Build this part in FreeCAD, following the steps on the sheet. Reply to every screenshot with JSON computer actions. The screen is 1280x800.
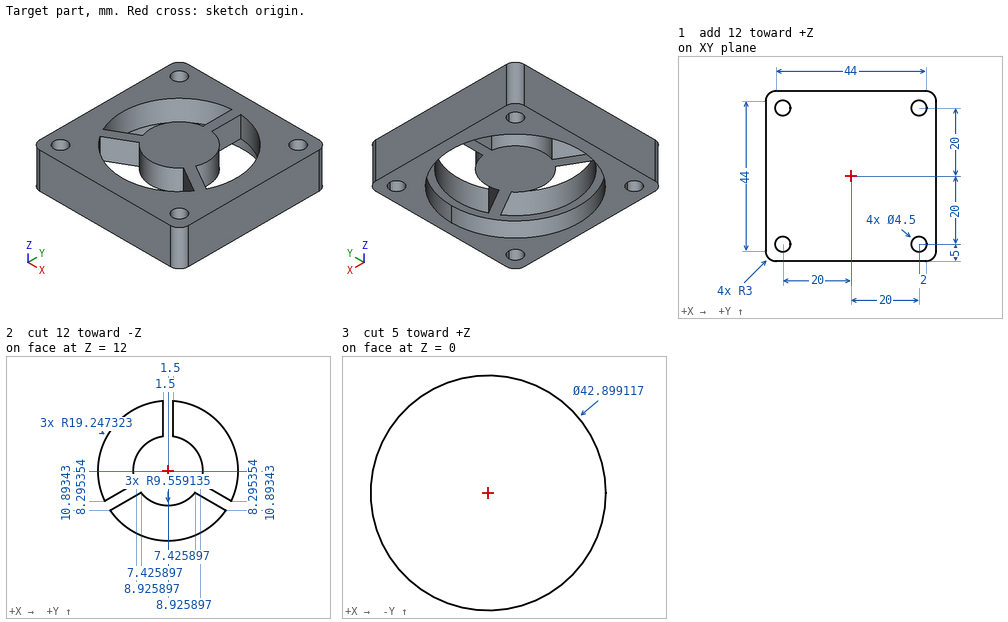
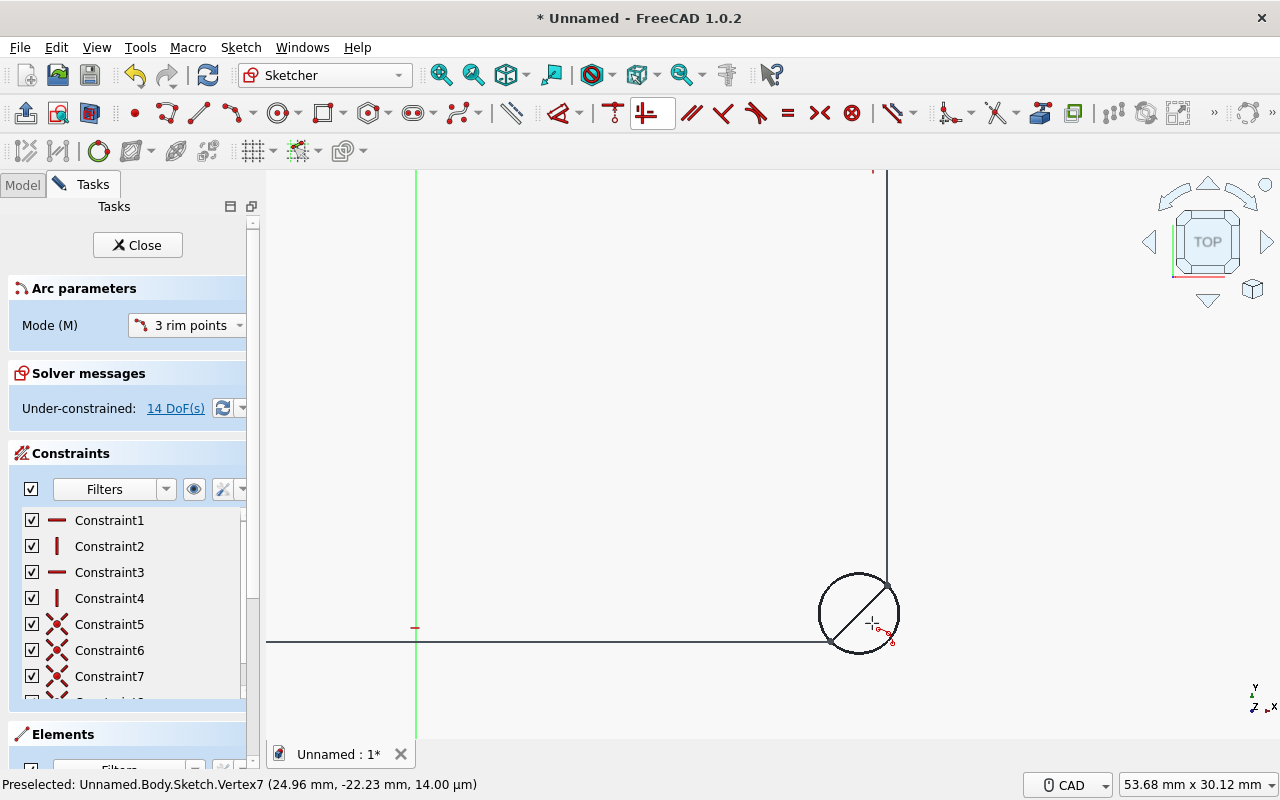
{"action": "left_click", "coordinate": [871, 621]}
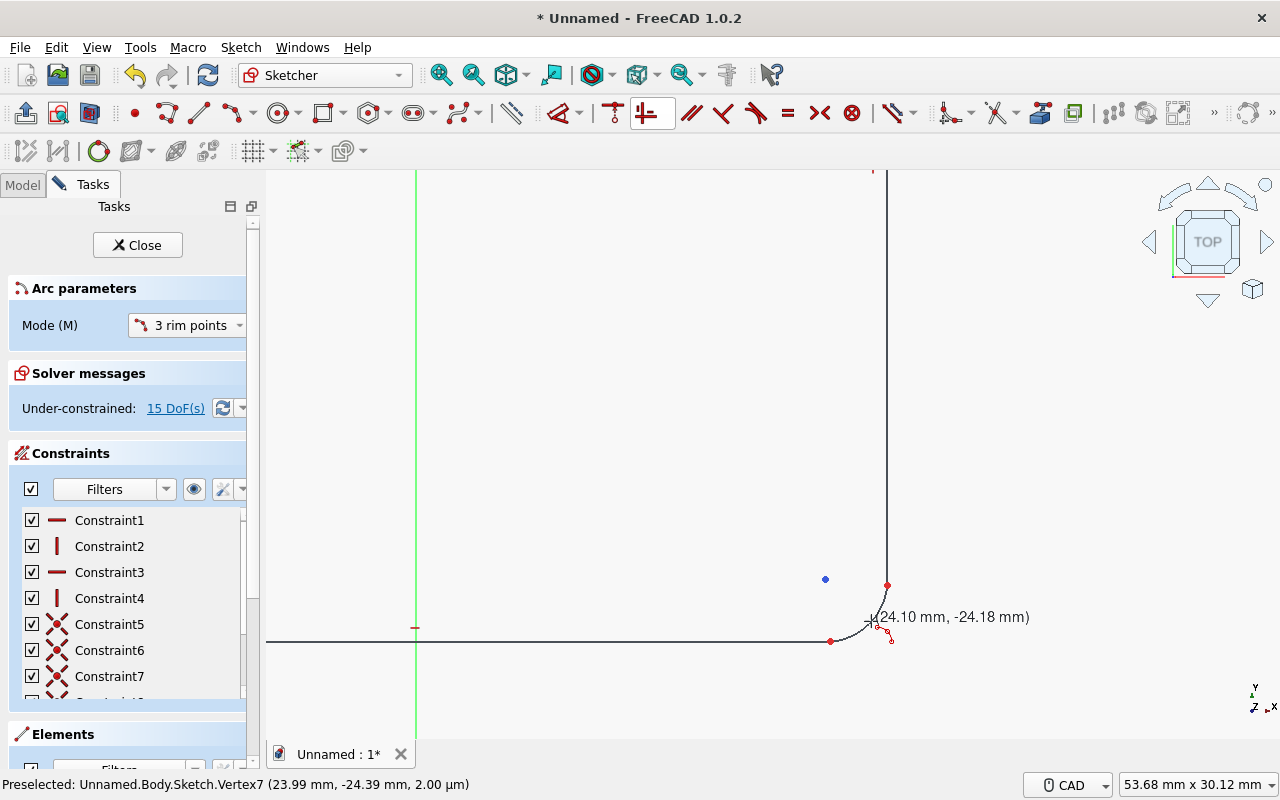
{"action": "scroll", "coordinate": [873, 623], "scroll_direction": "down", "scroll_amount": 5}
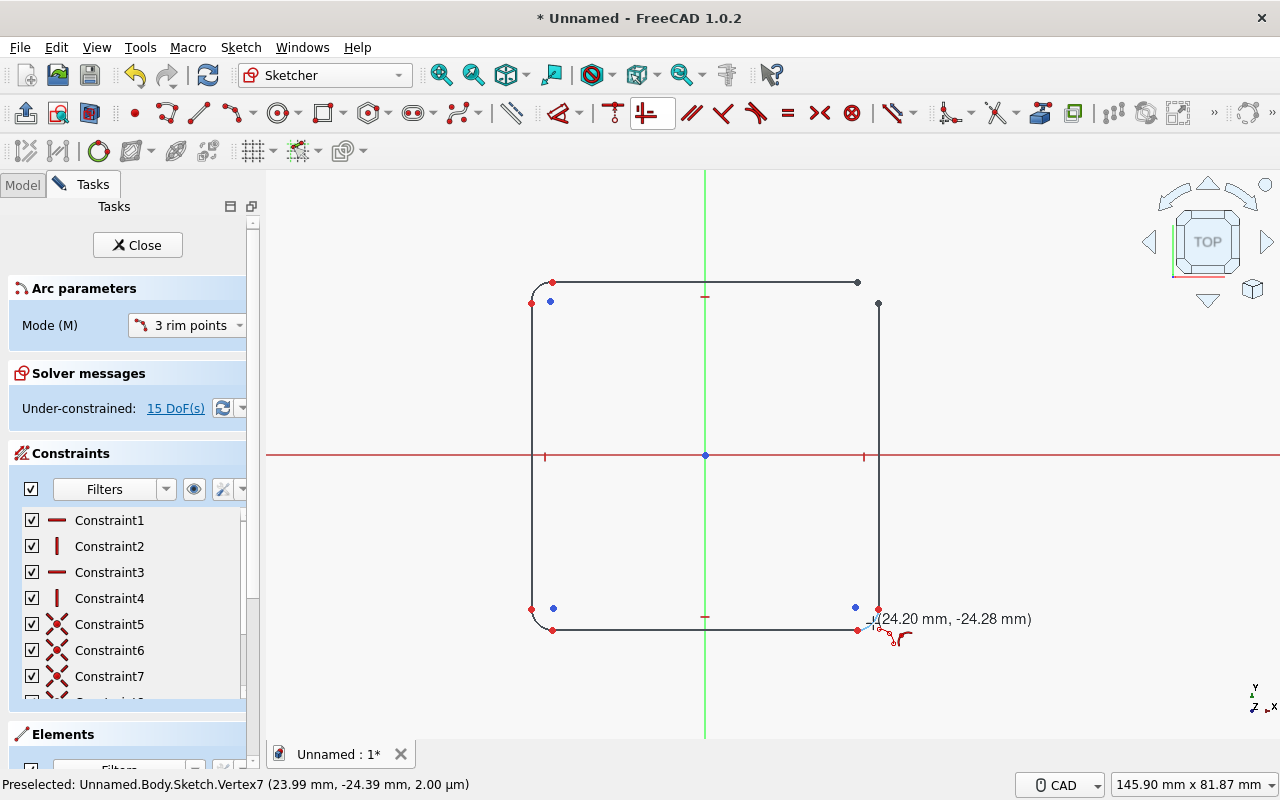
{"action": "left_click", "coordinate": [879, 303]}
{"action": "left_click", "coordinate": [858, 282]}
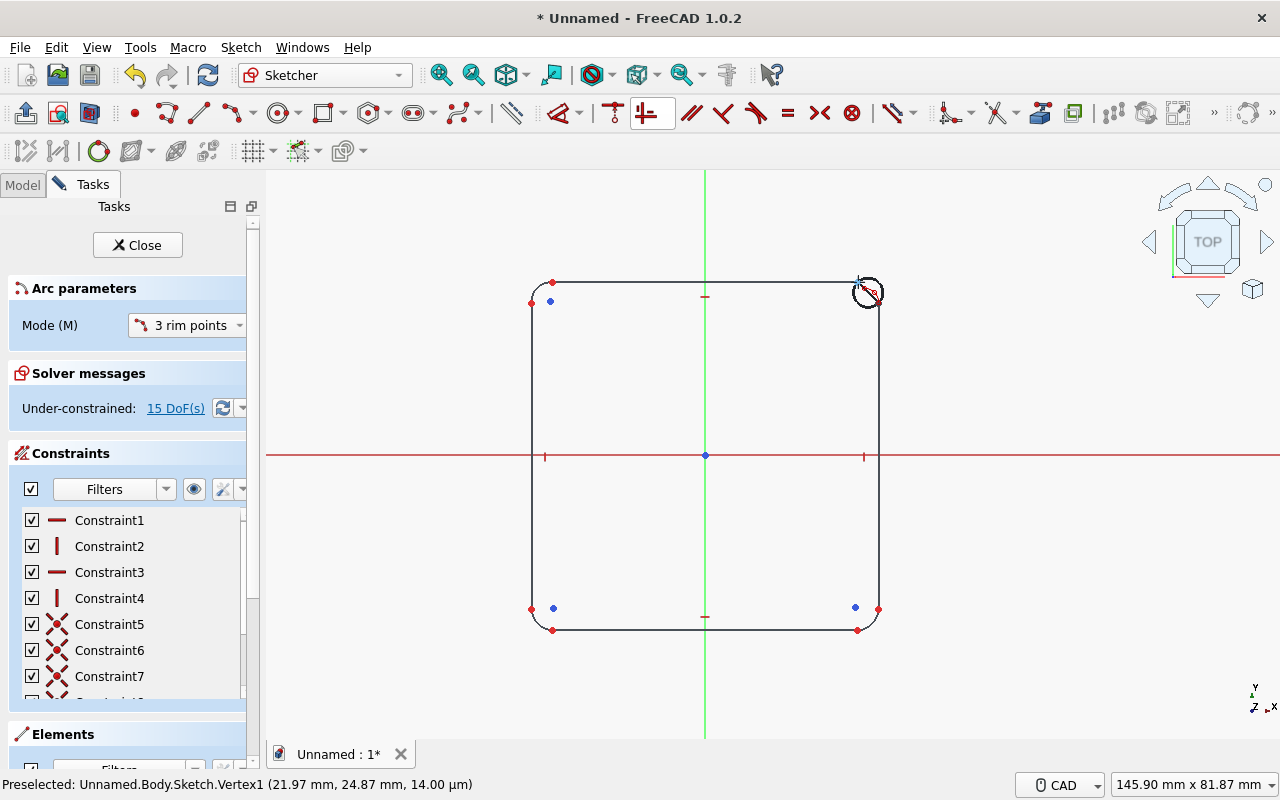
{"action": "scroll", "coordinate": [873, 287], "scroll_direction": "up", "scroll_amount": 5}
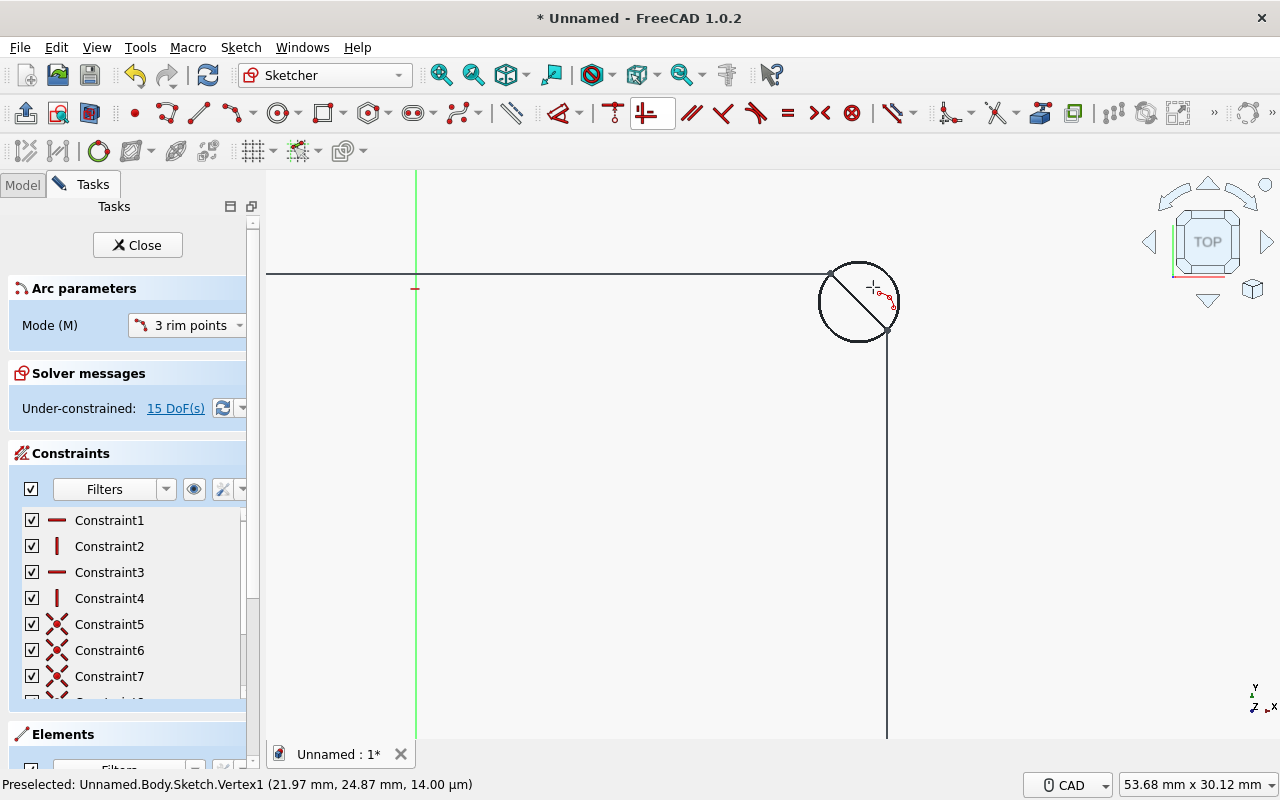
{"action": "left_click", "coordinate": [871, 288]}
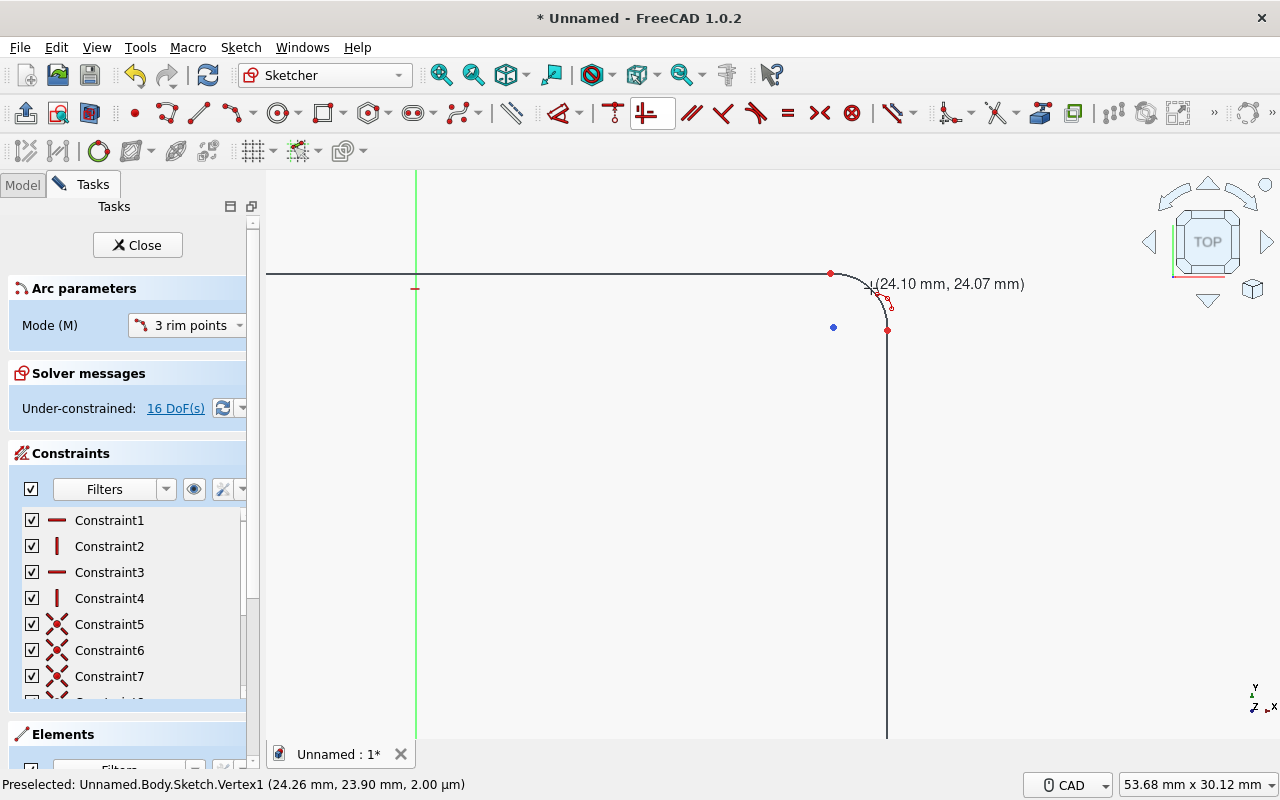
{"action": "left_click", "coordinate": [278, 114]}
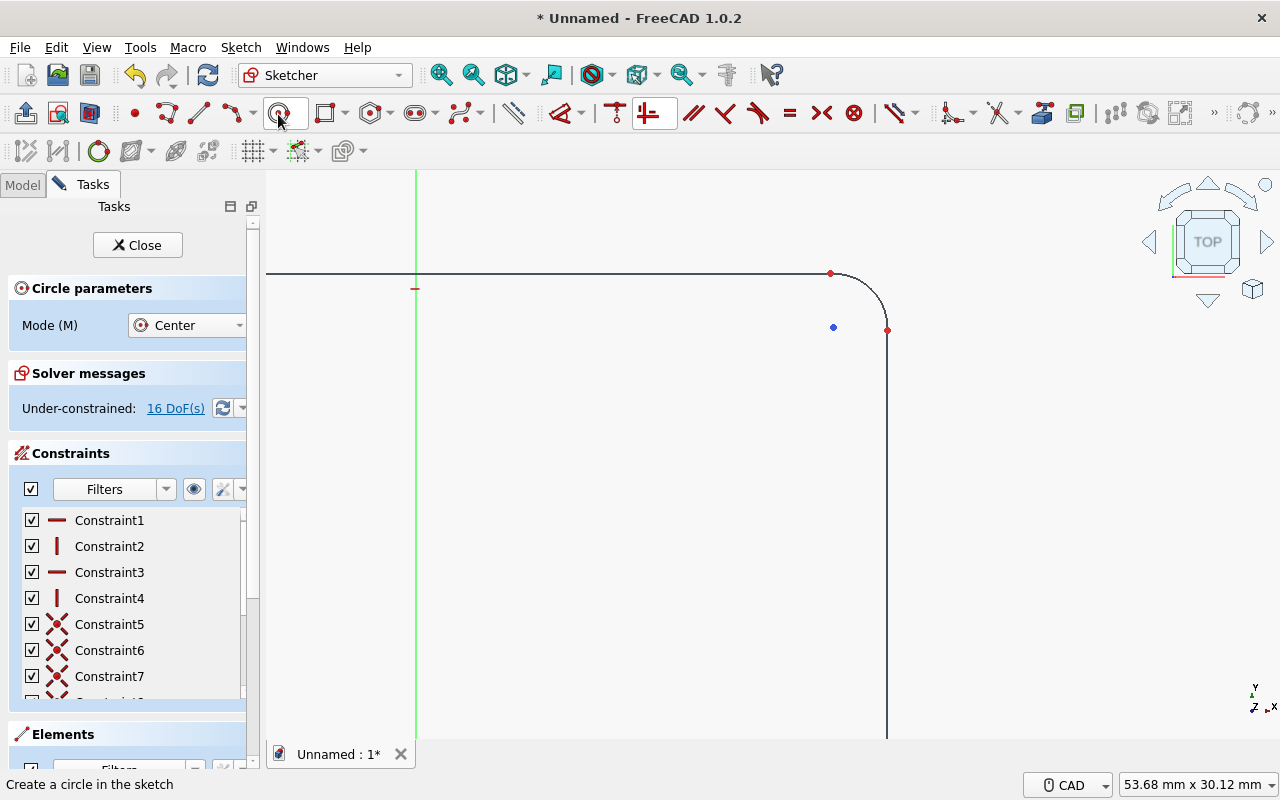
{"action": "scroll", "coordinate": [873, 286], "scroll_direction": "down", "scroll_amount": 5}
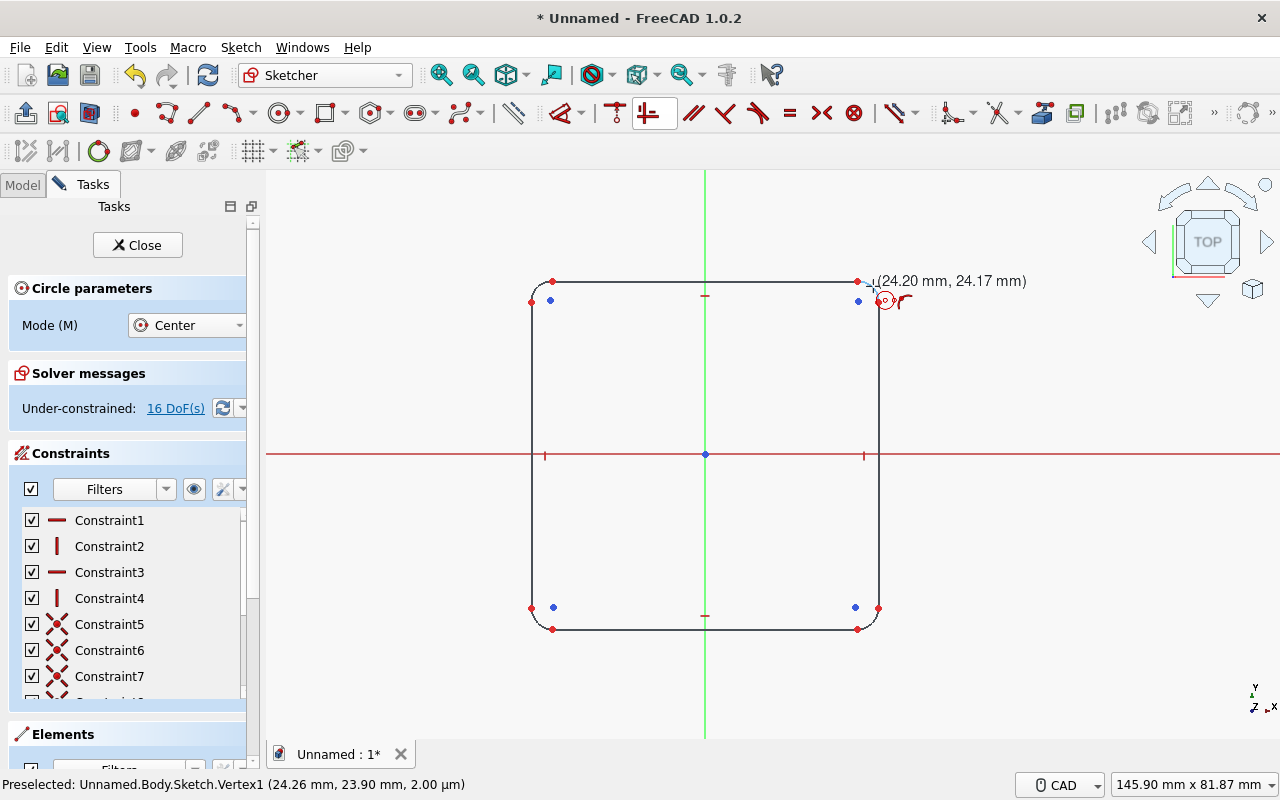
{"action": "scroll", "coordinate": [844, 593], "scroll_direction": "up", "scroll_amount": 2}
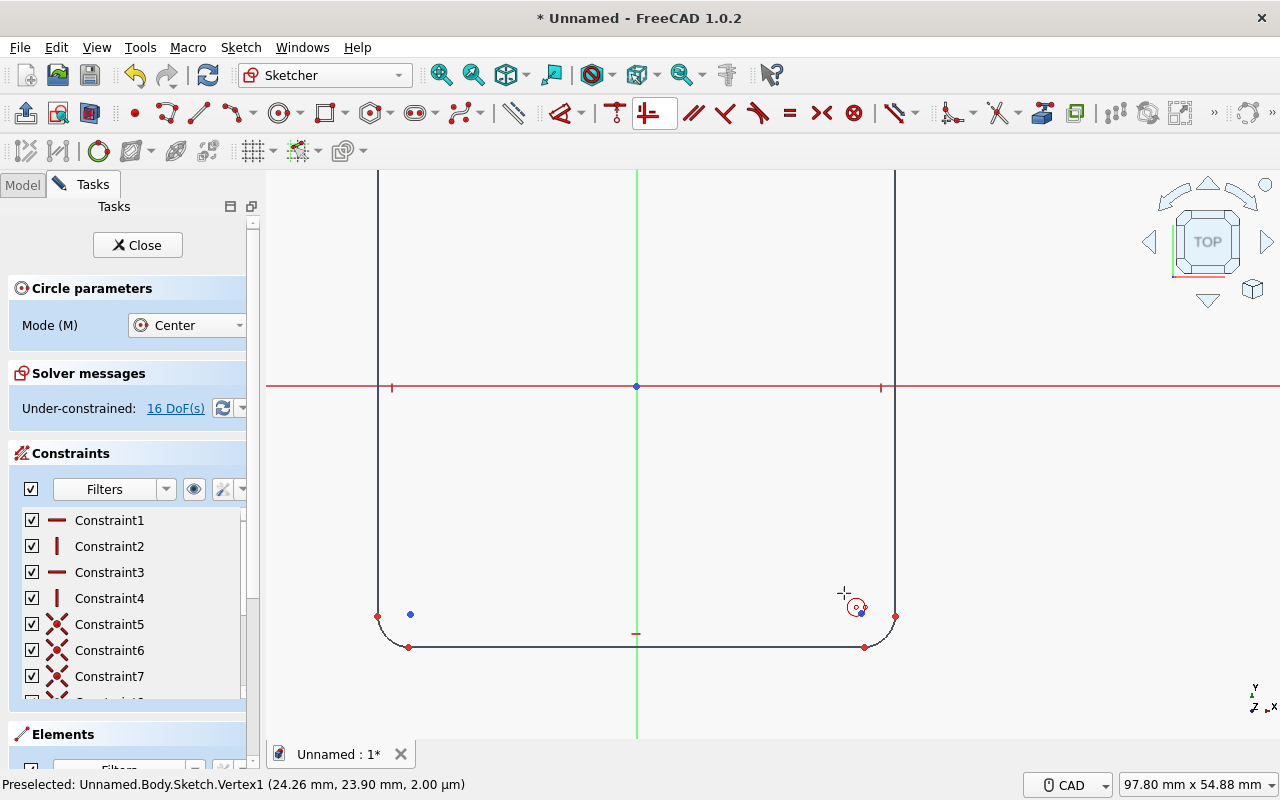
{"action": "left_click", "coordinate": [844, 593]}
{"action": "left_click", "coordinate": [860, 577]}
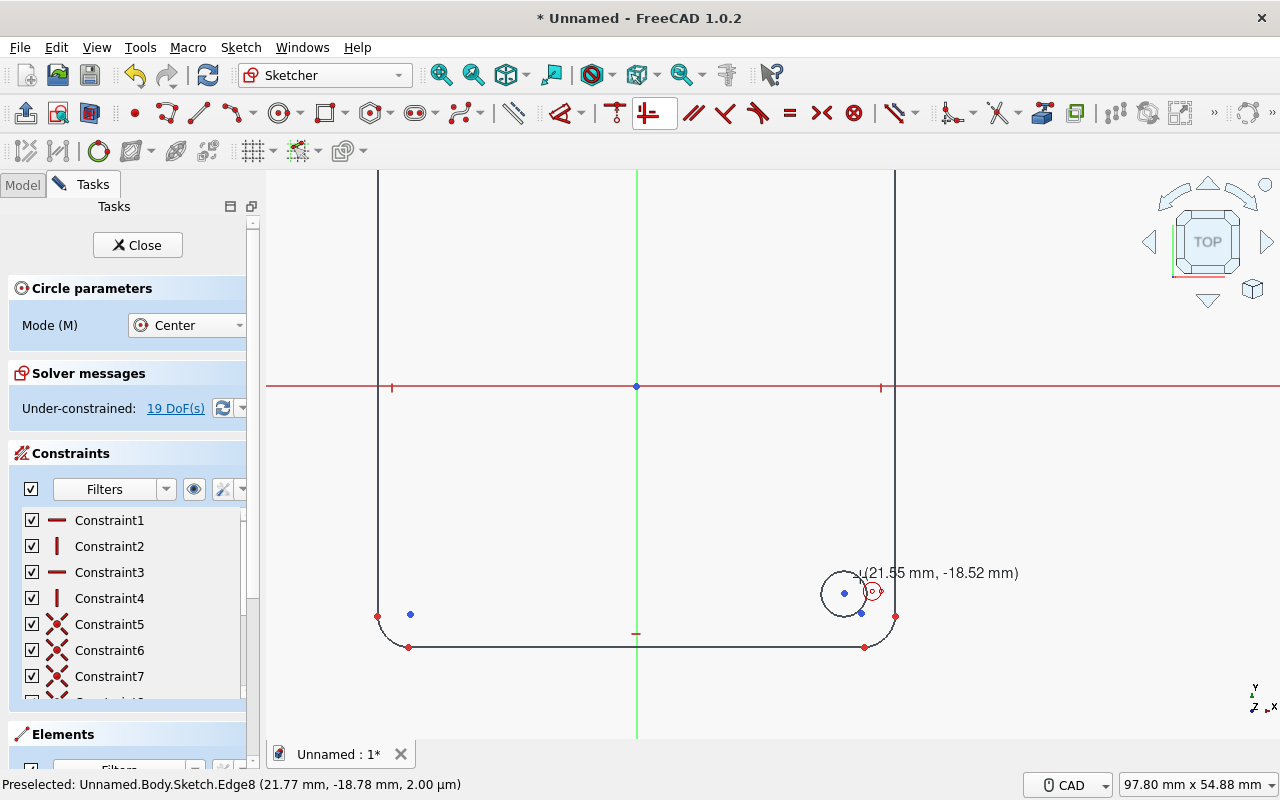
{"action": "left_click", "coordinate": [429, 593]}
{"action": "left_click", "coordinate": [446, 577]}